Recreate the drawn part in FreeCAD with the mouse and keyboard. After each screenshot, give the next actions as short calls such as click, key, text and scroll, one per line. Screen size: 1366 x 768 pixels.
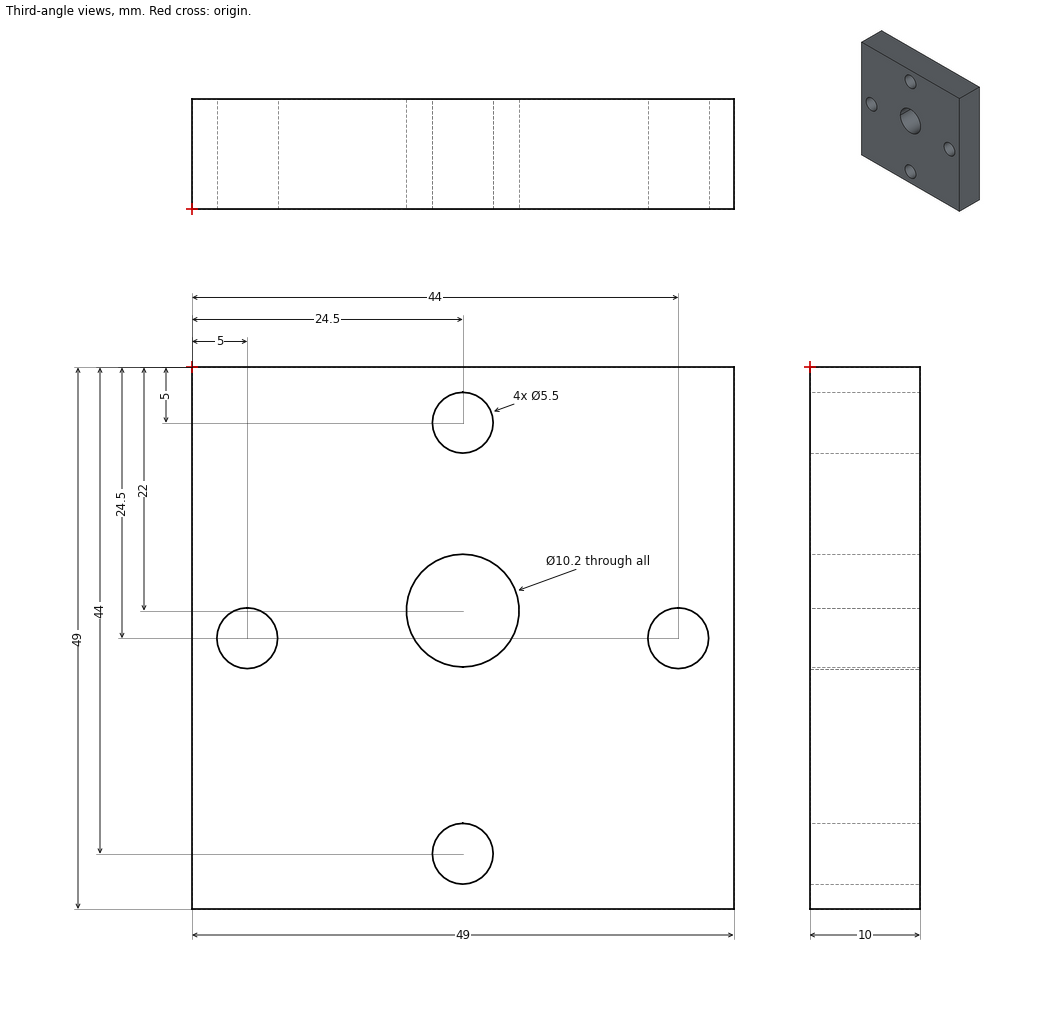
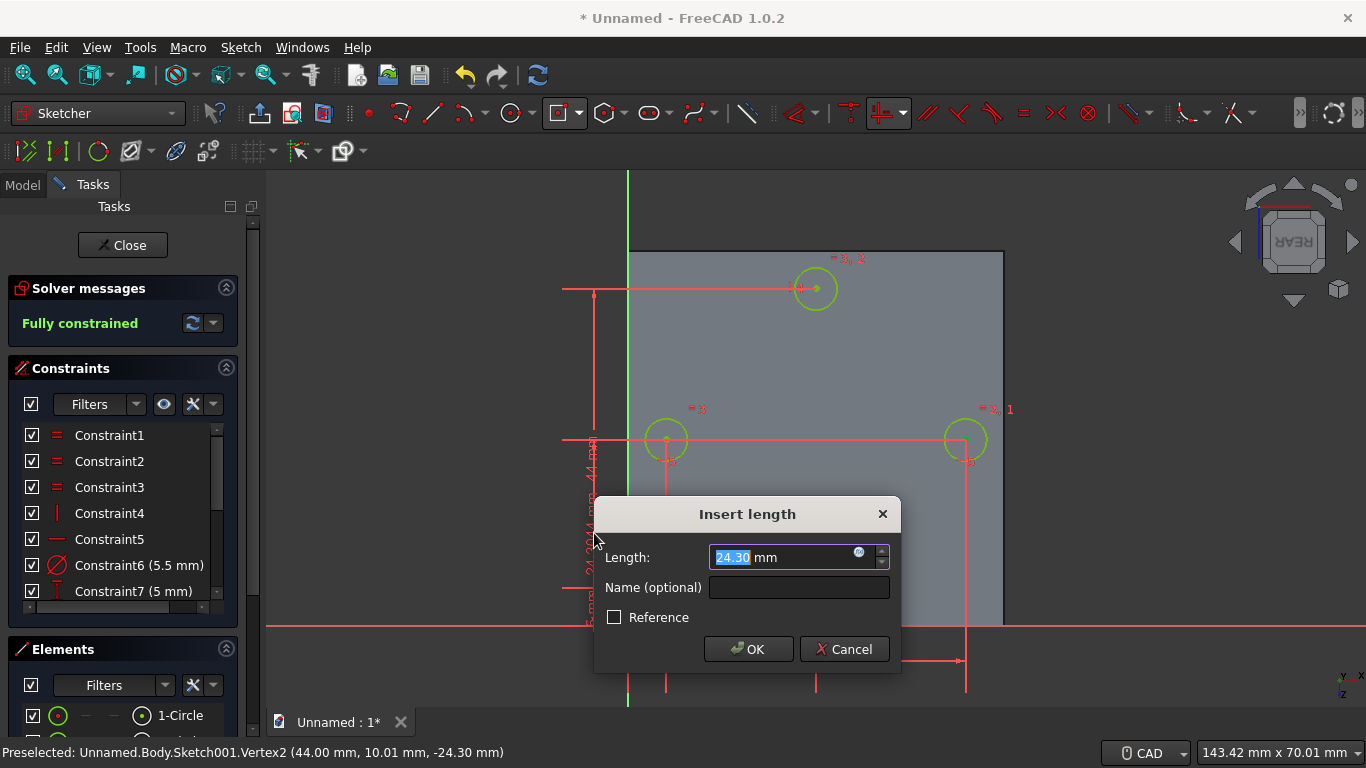
text(24.5)
key(Return)
key(Escape)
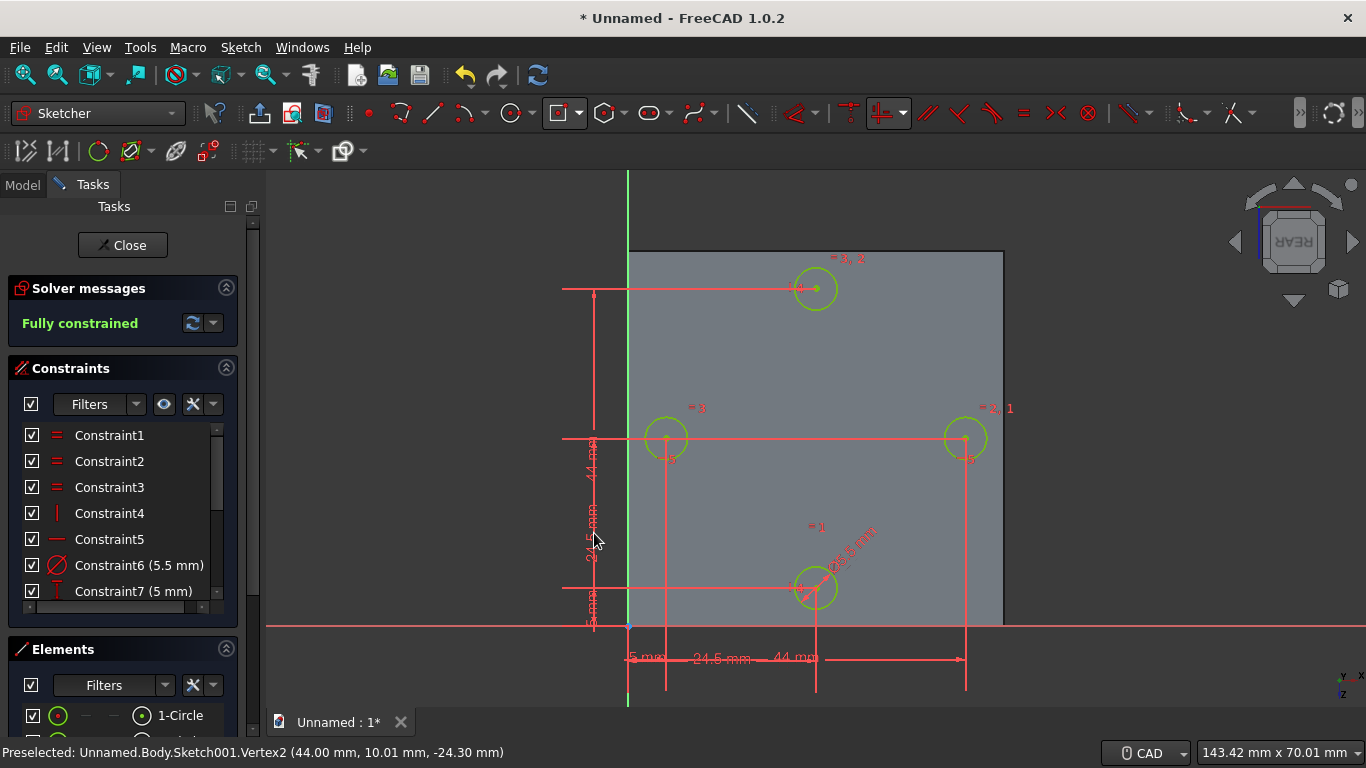
click(123, 245)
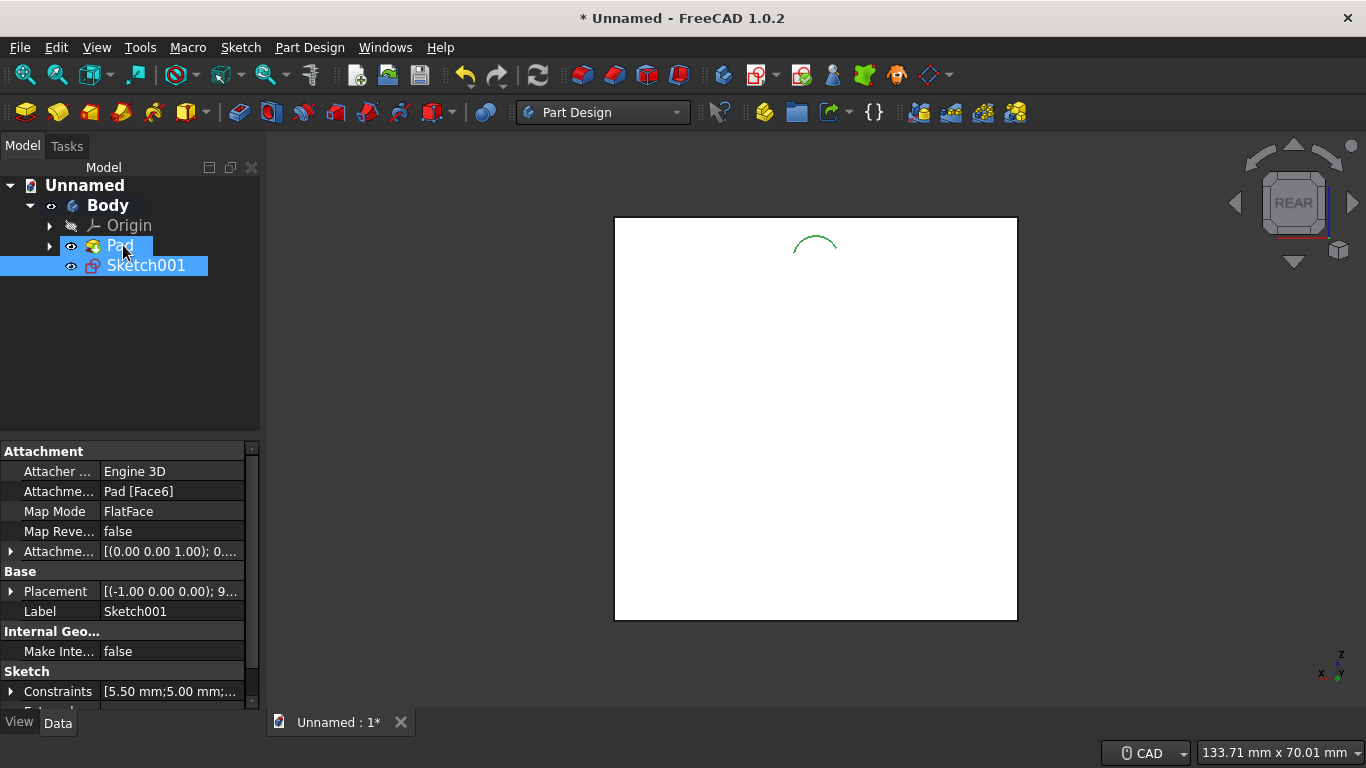
click(240, 112)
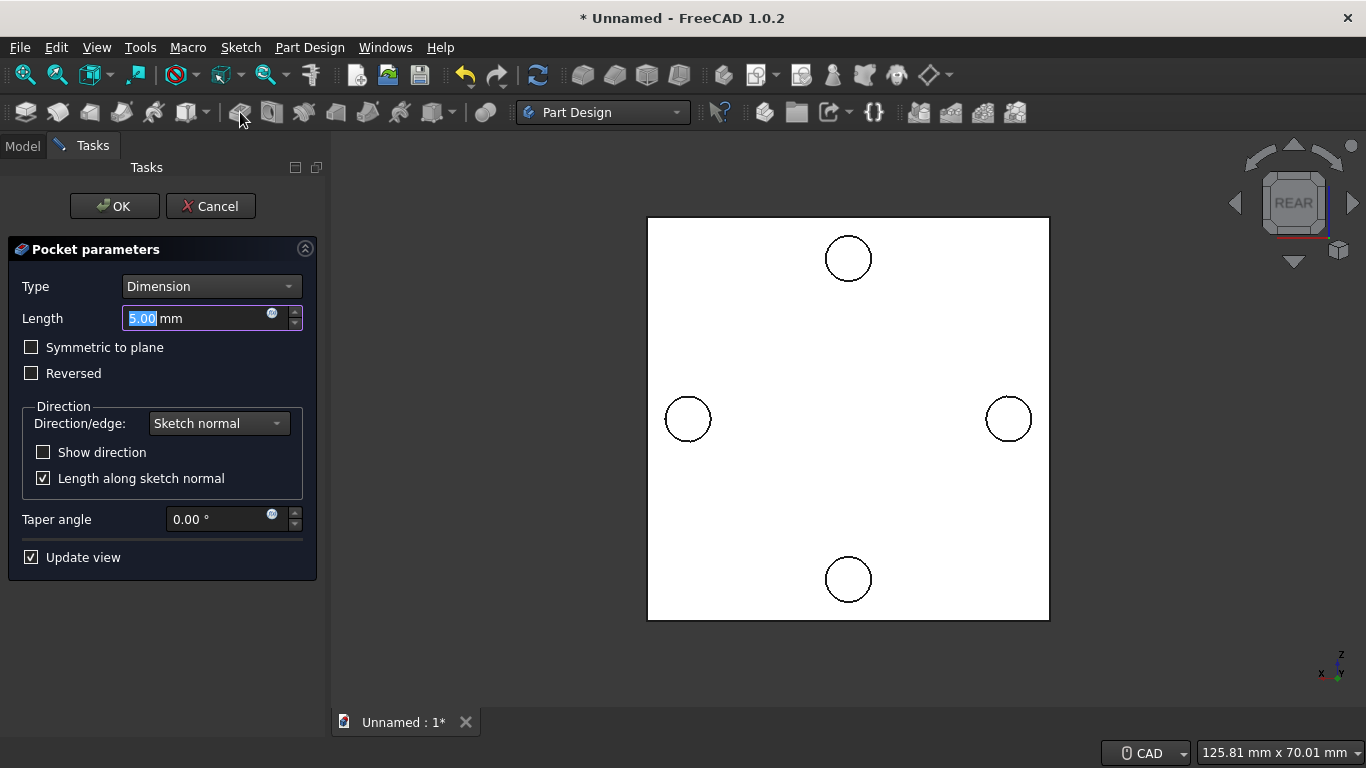
click(212, 286)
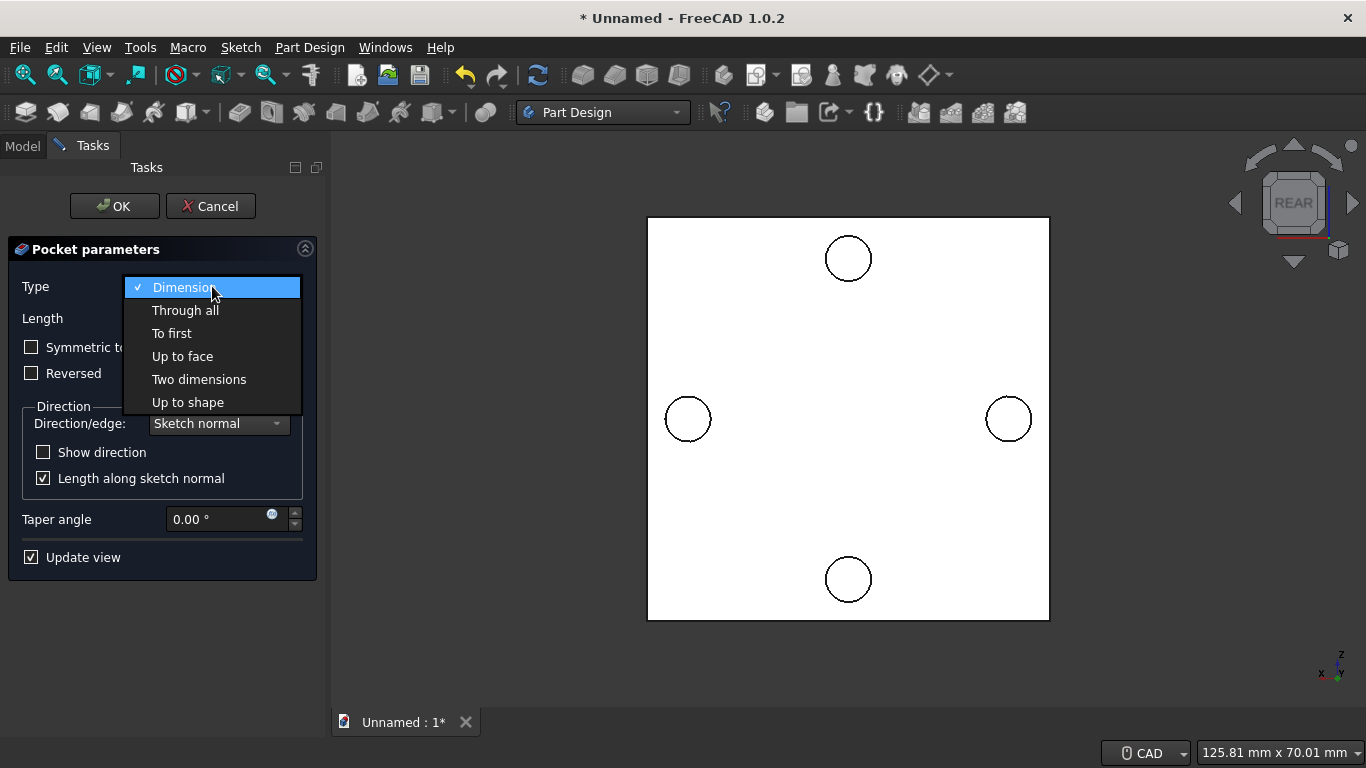
click(212, 310)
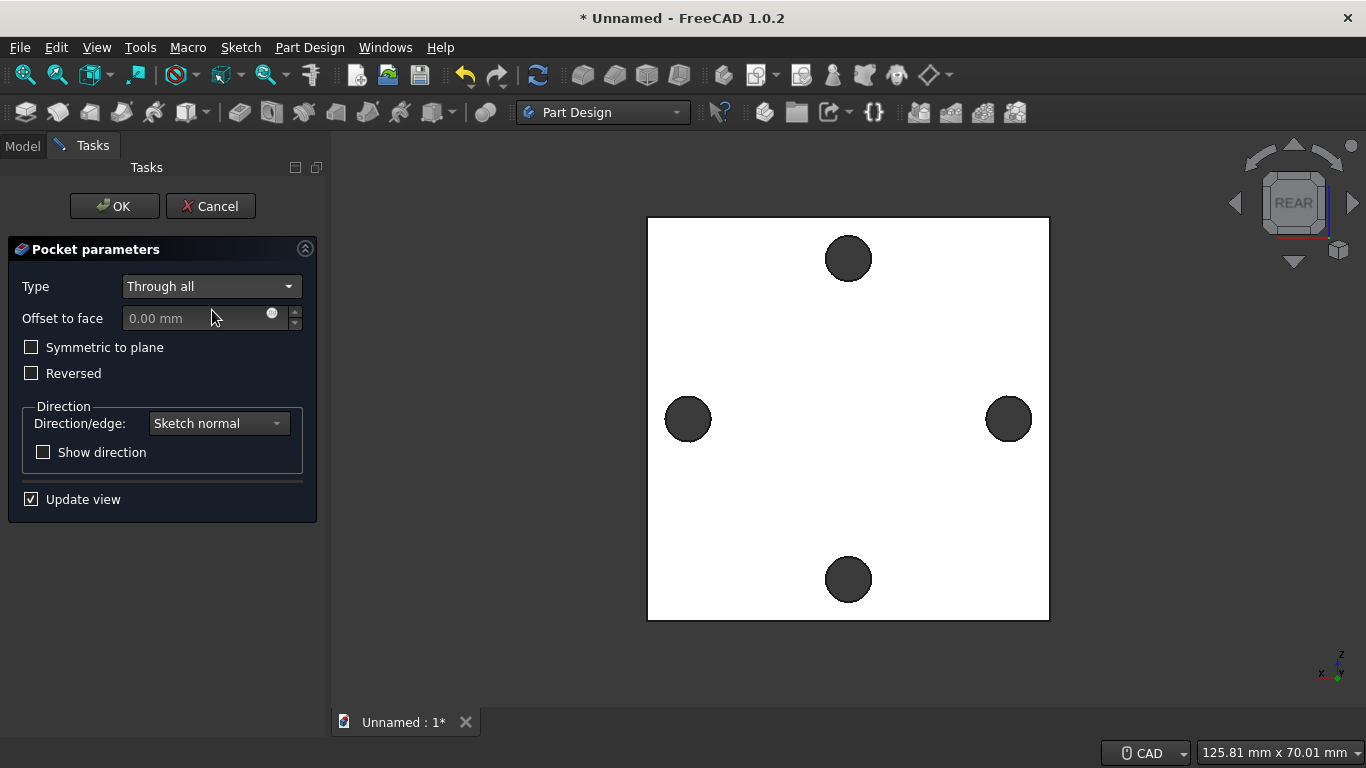
click(115, 206)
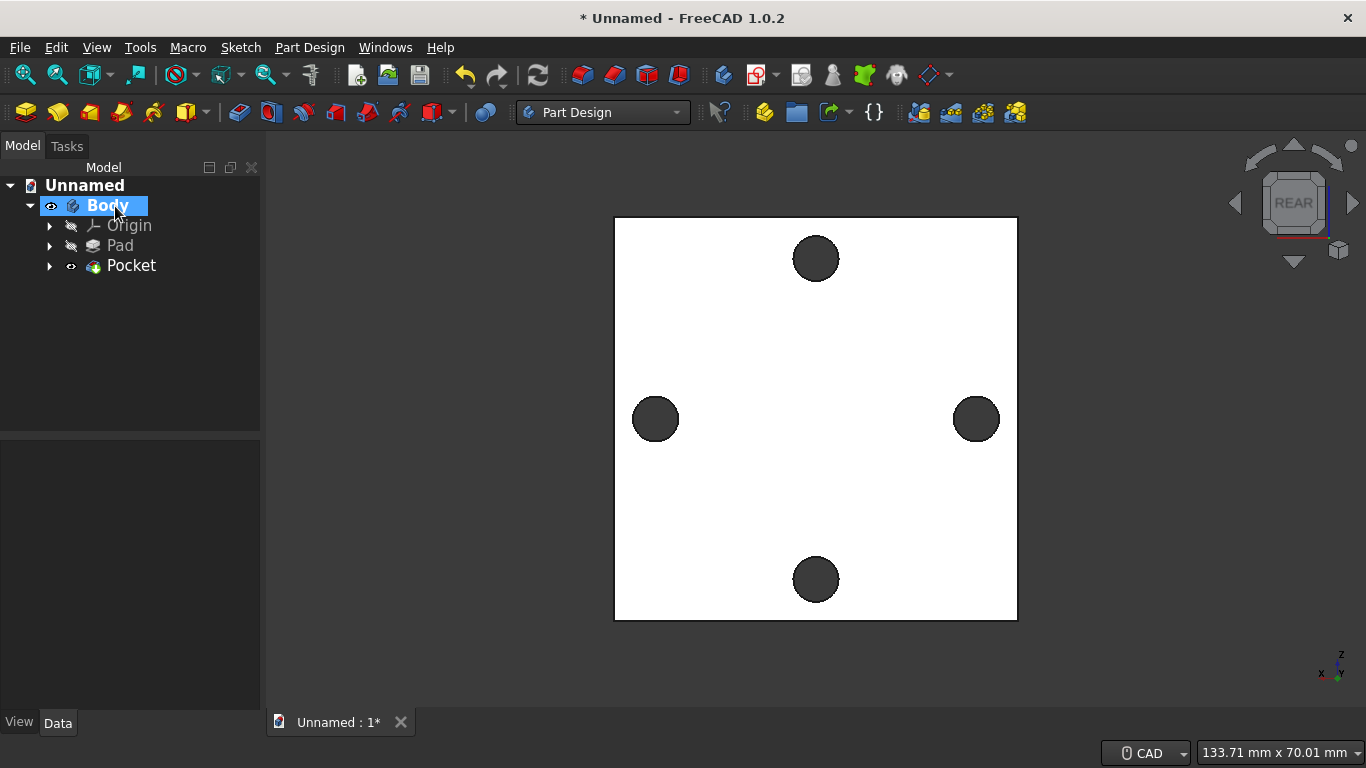
click(816, 418)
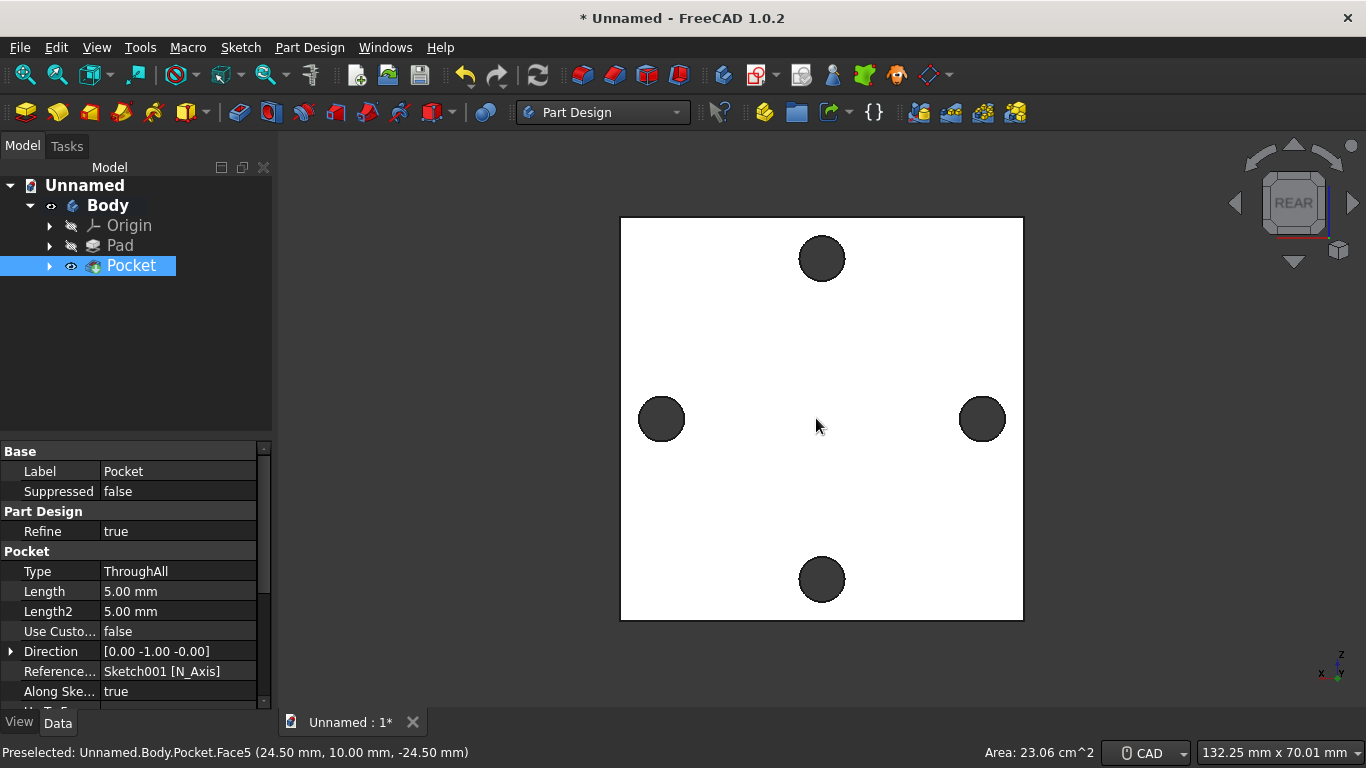
click(756, 76)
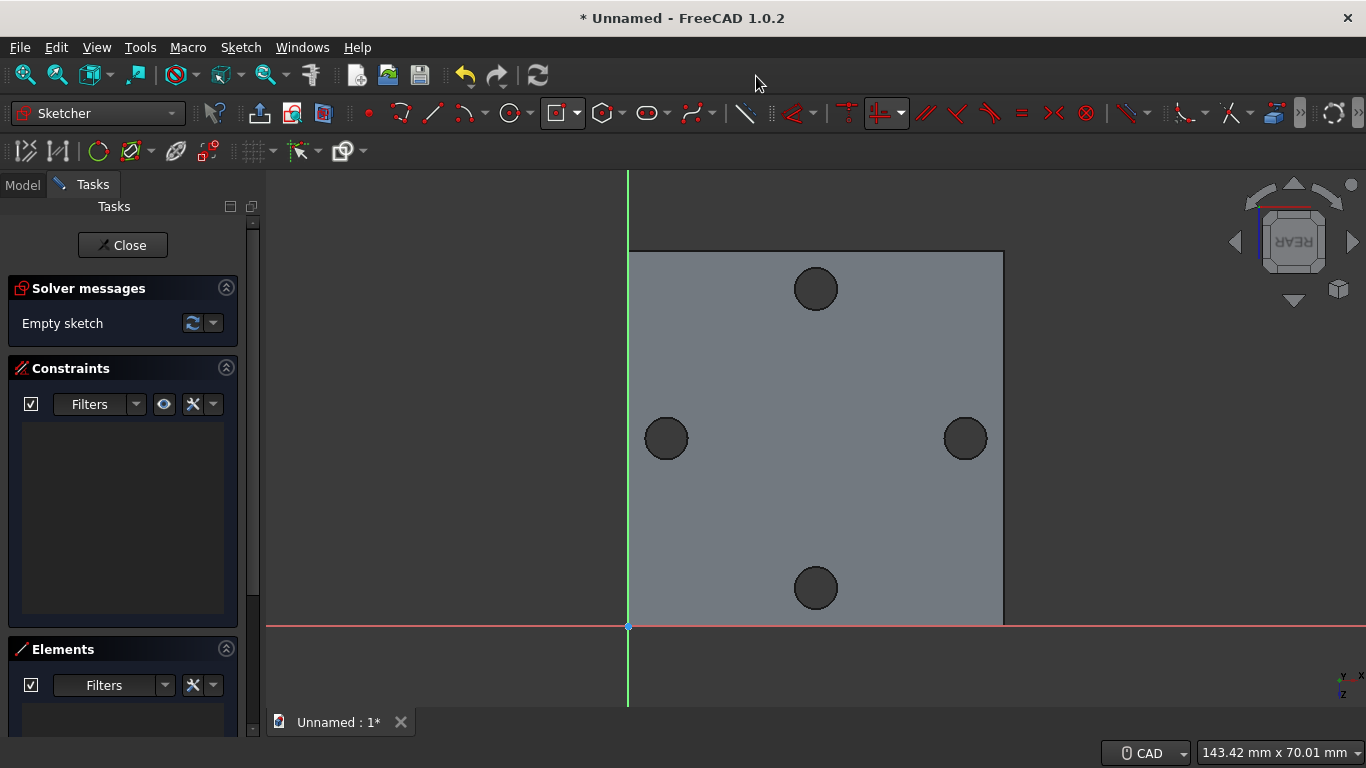
scroll(838, 464, up, 7)